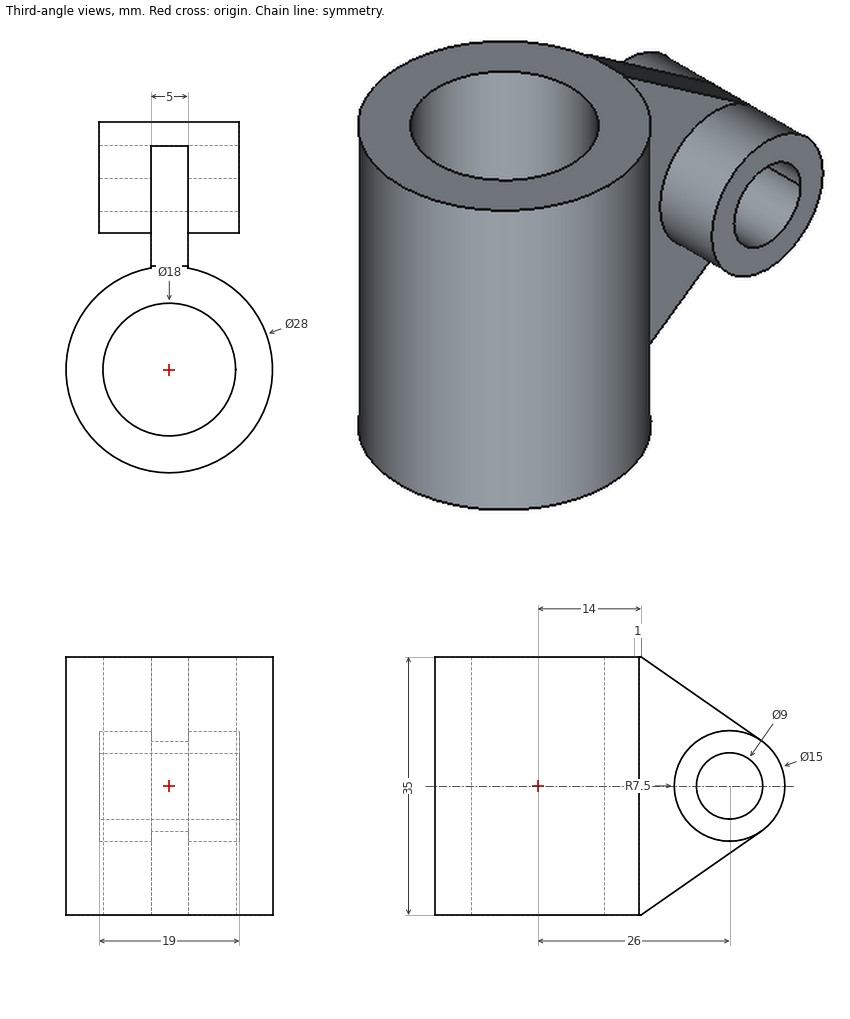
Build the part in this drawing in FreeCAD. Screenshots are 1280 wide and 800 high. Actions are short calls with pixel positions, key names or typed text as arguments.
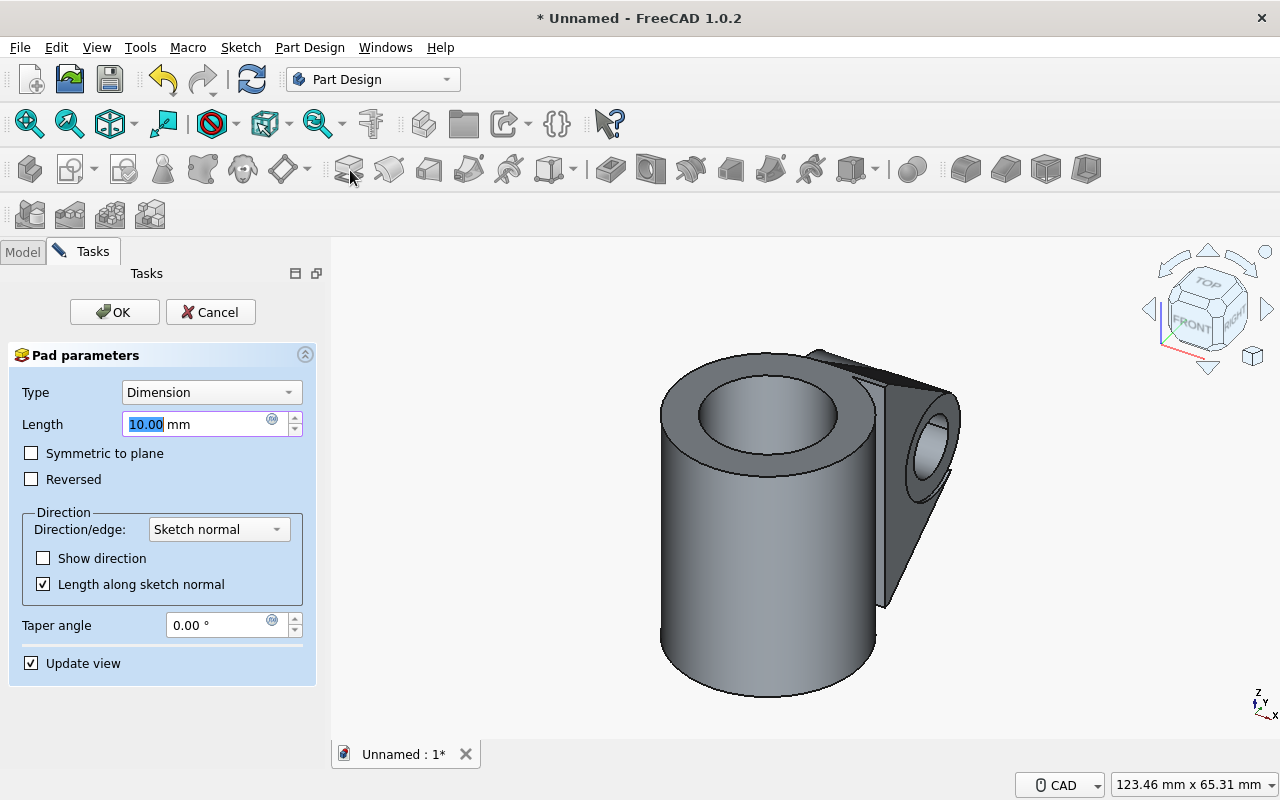
text(5)
key(Tab)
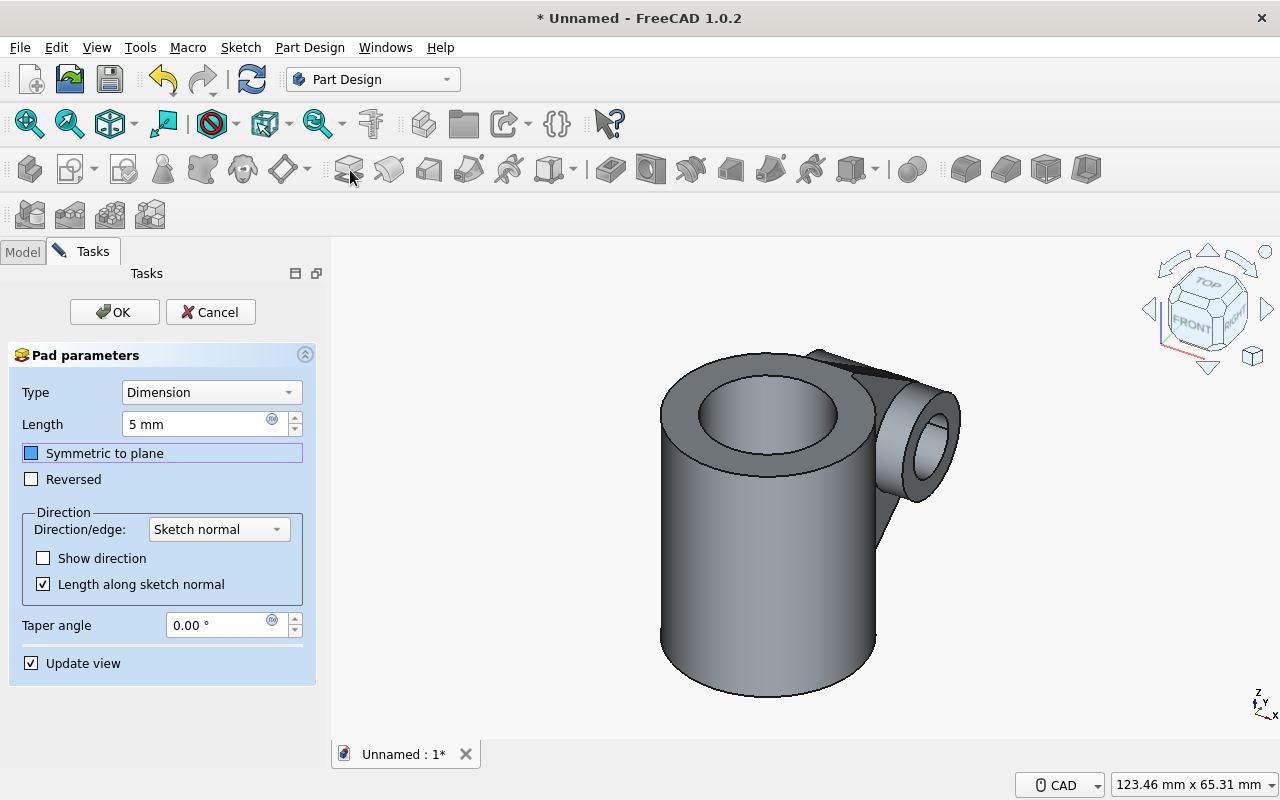
click(30, 453)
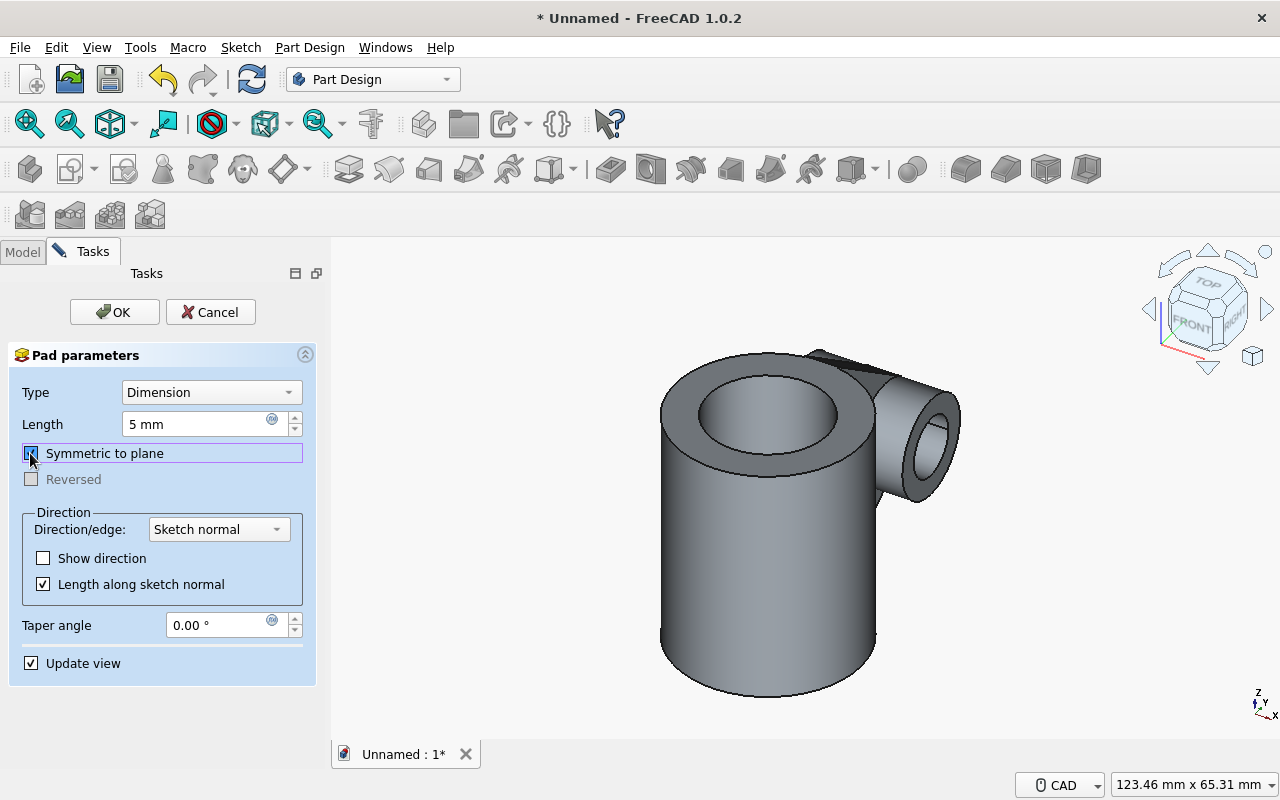
click(115, 312)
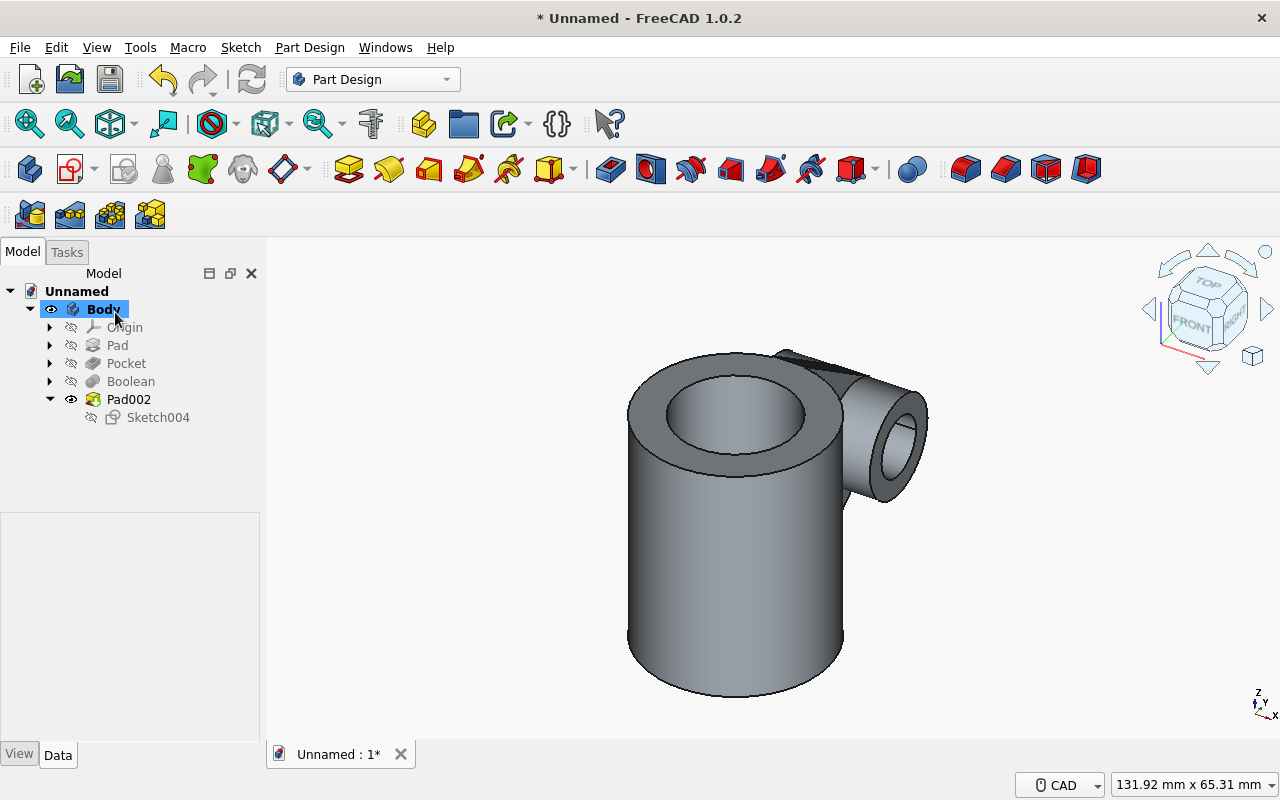
key(0)